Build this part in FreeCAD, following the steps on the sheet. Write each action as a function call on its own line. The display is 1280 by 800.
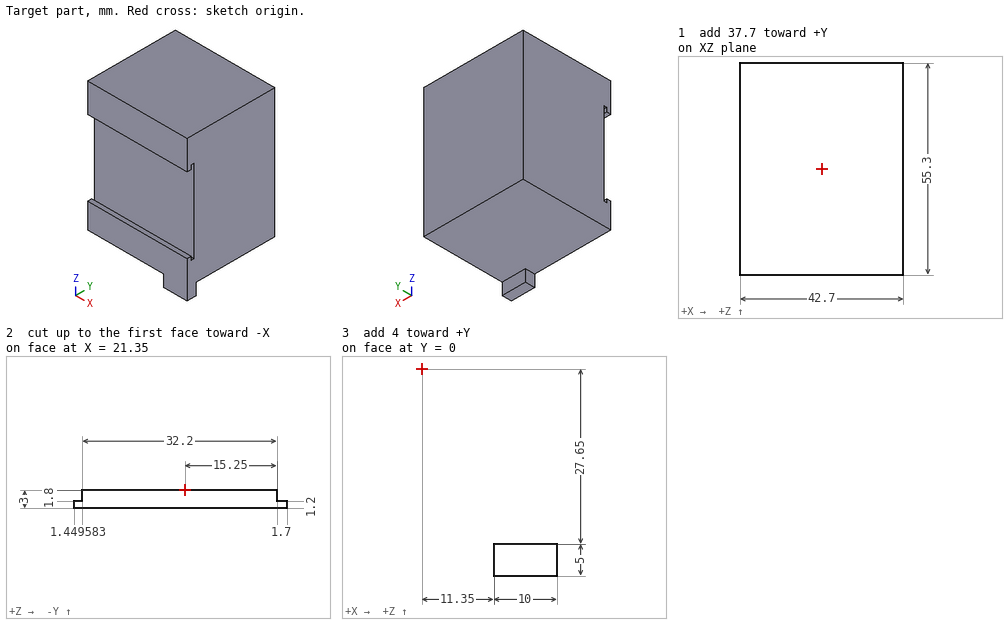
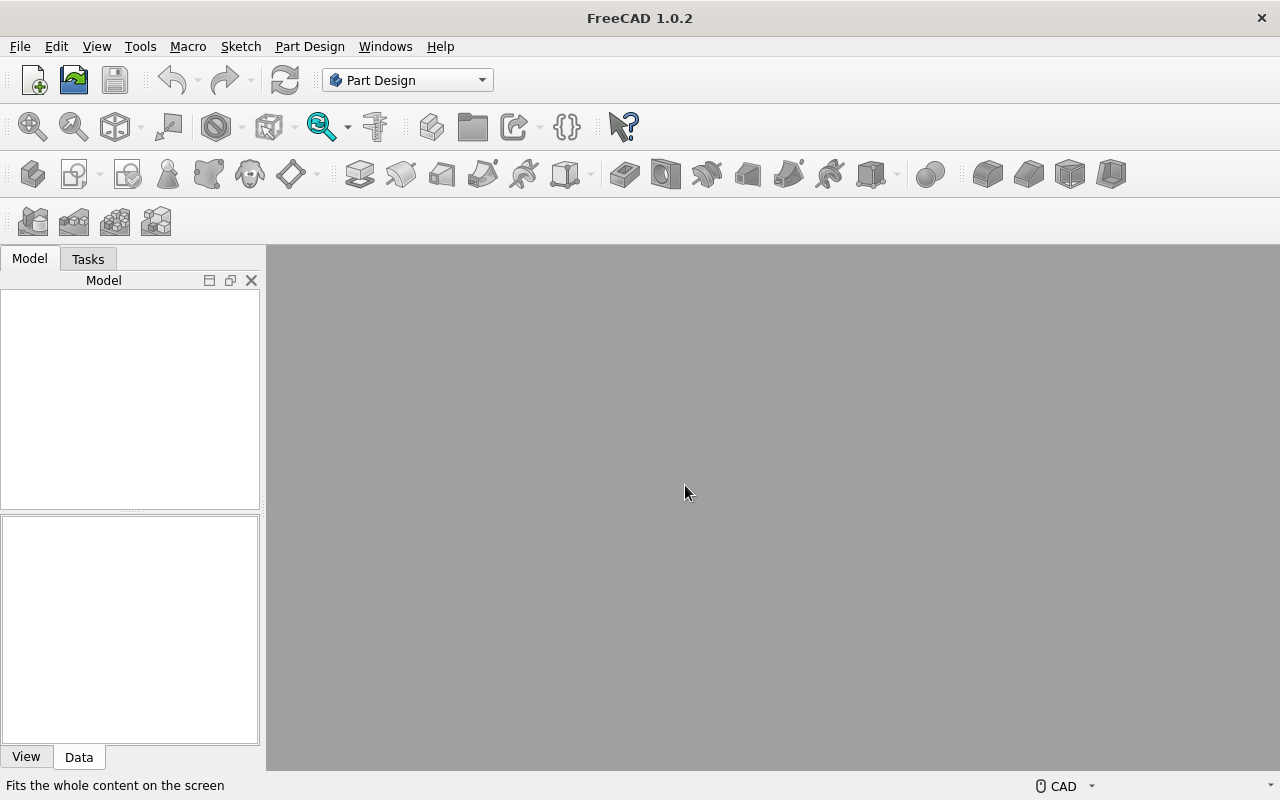
key(ctrl+n)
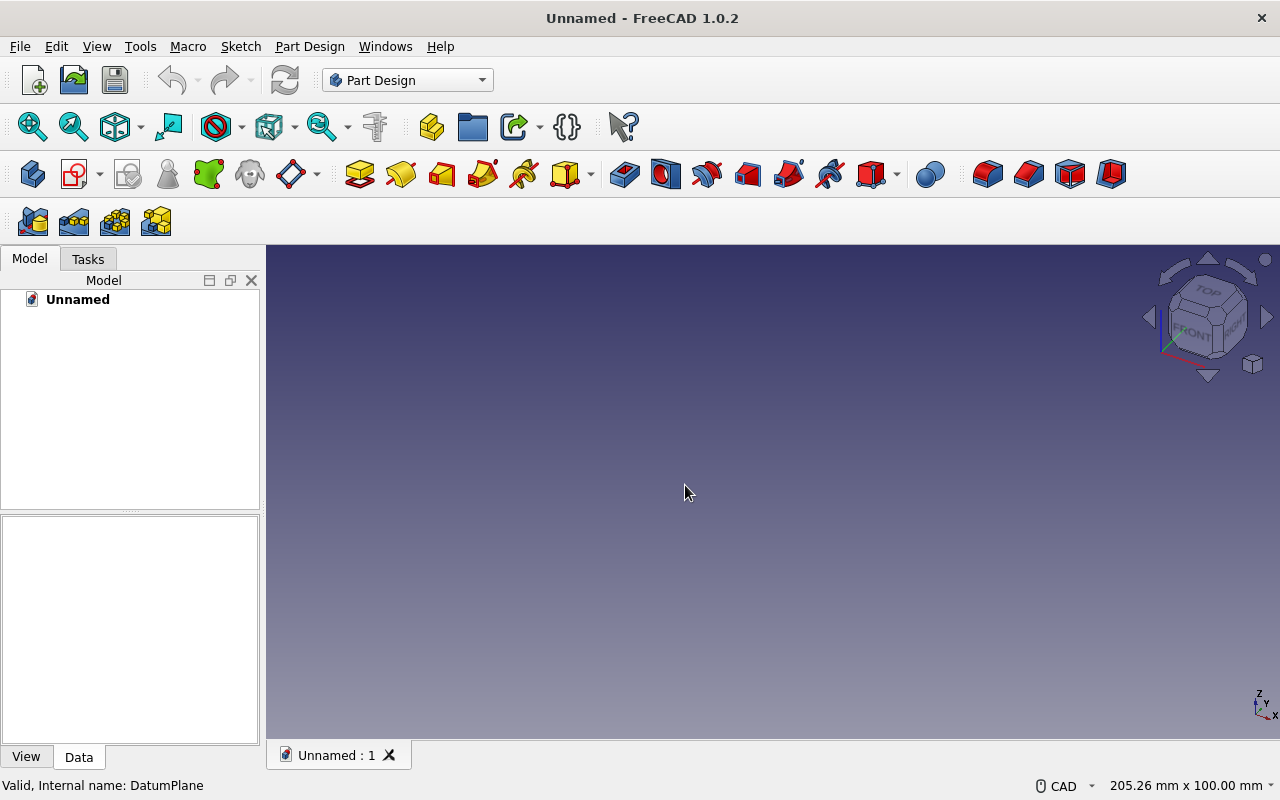
click(74, 174)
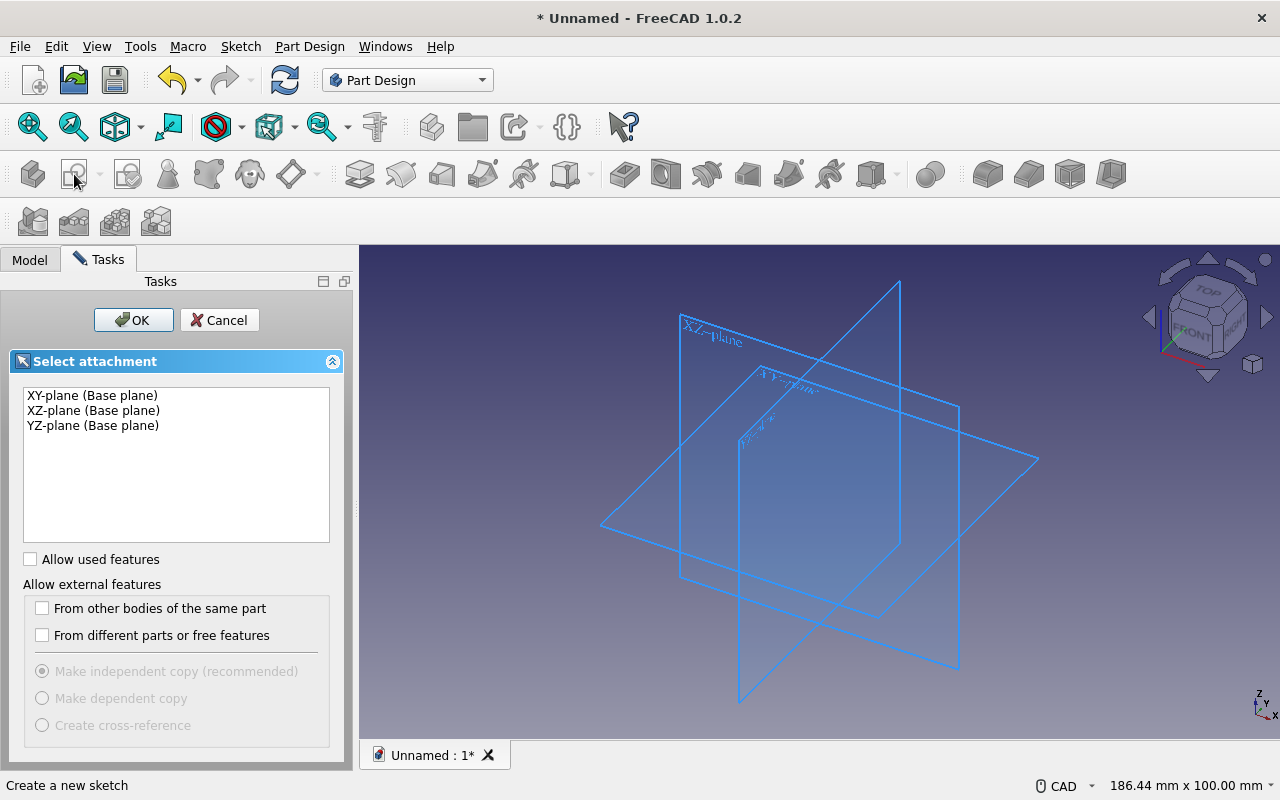
click(84, 410)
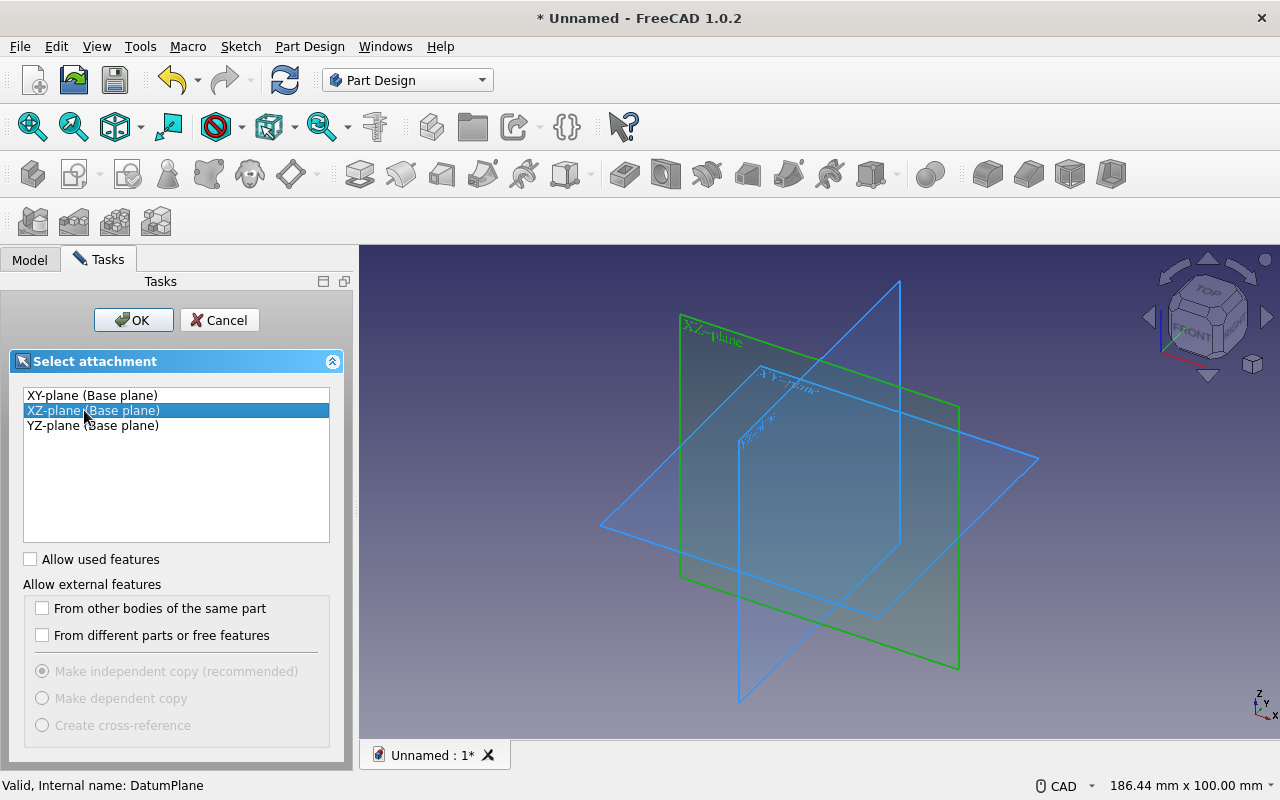
click(134, 320)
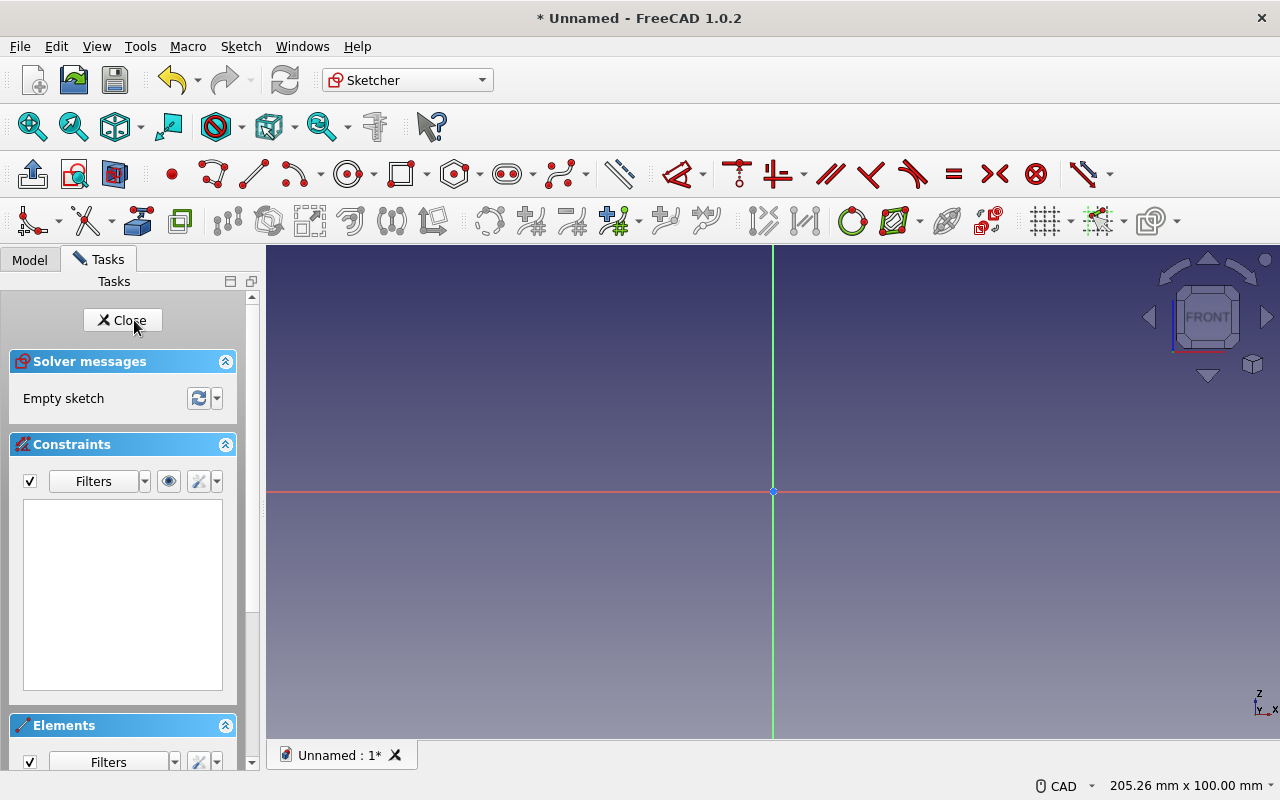
key(g)
key(v)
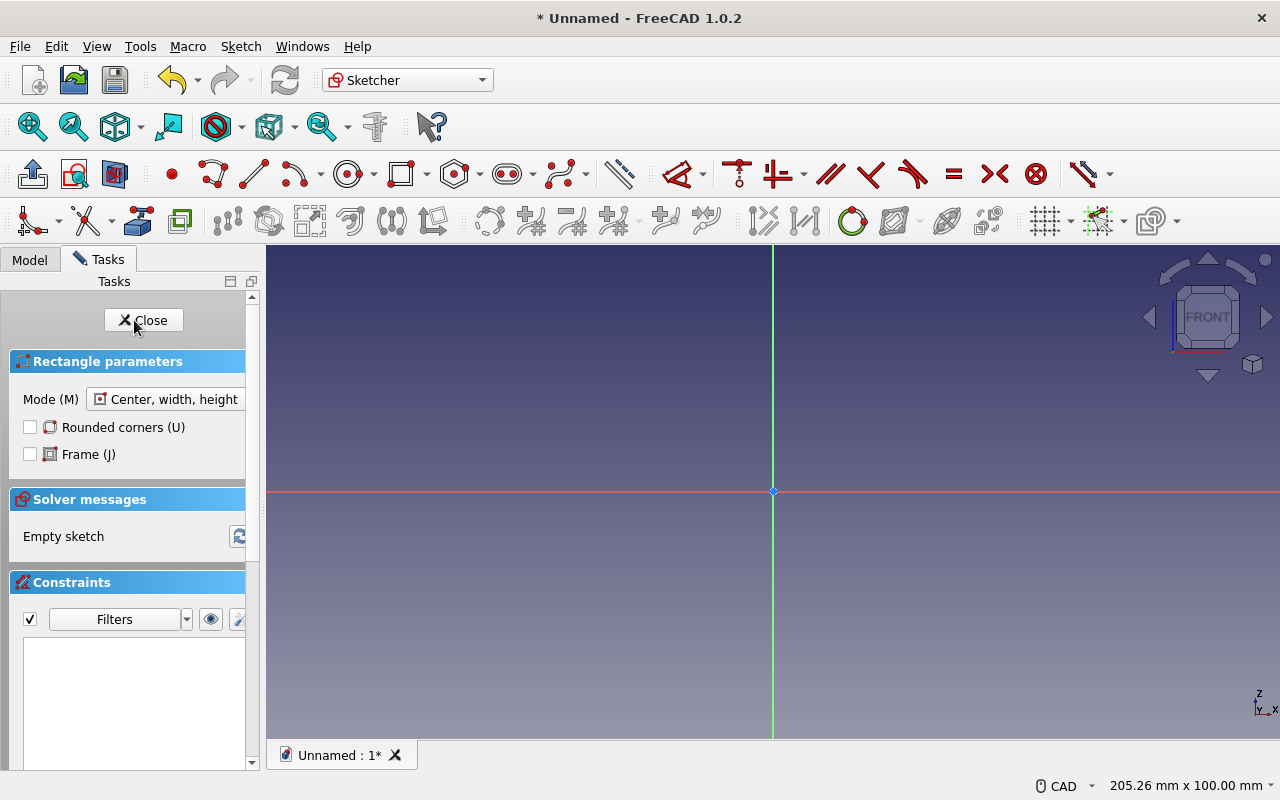
click(773, 492)
move(878, 355)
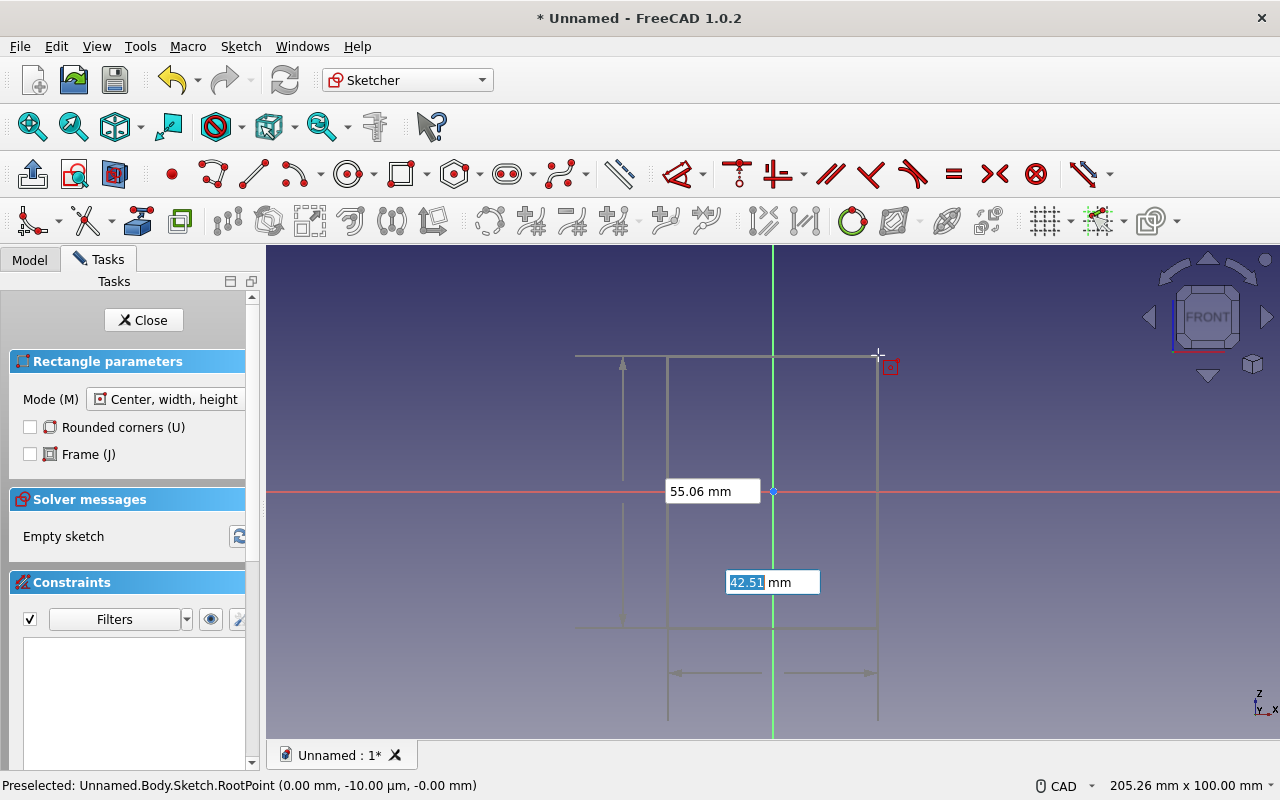
text(42.7)
key(Tab)
text(55.3)
key(Return)
key(Escape)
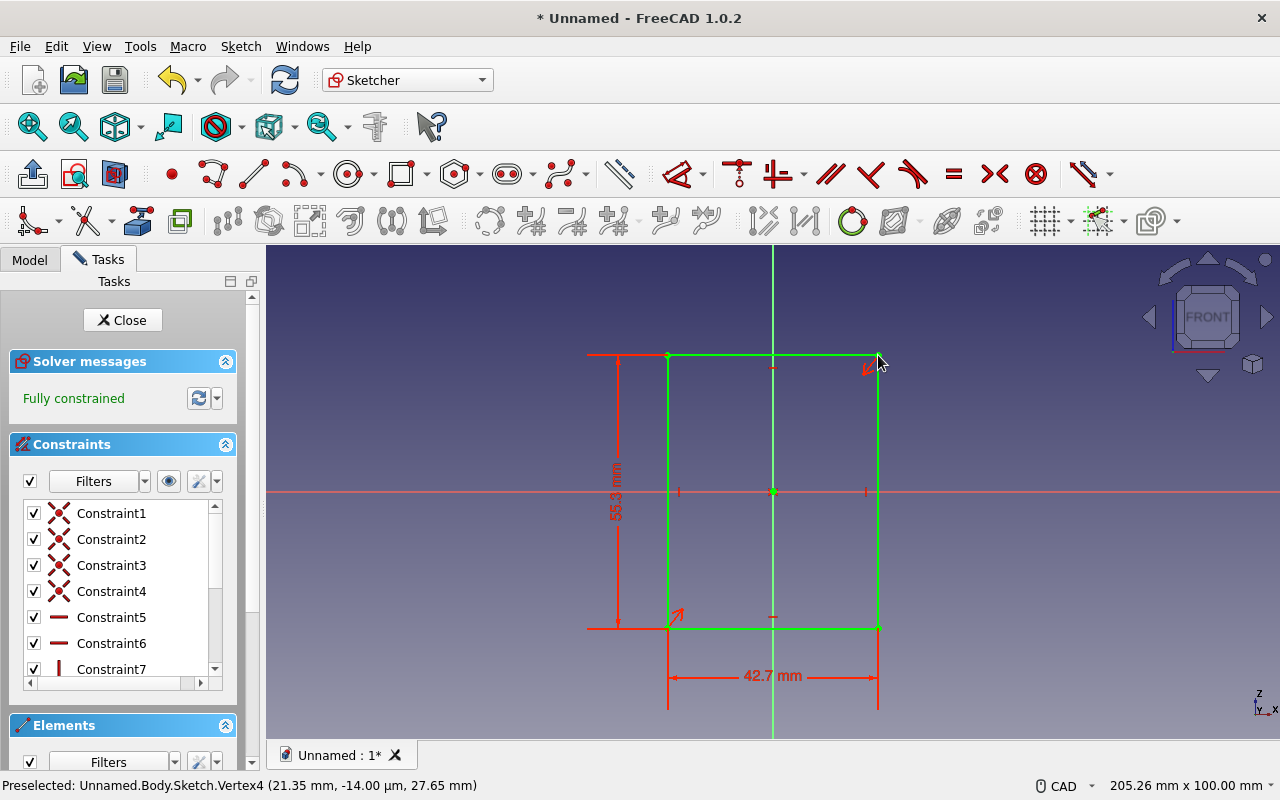
click(123, 320)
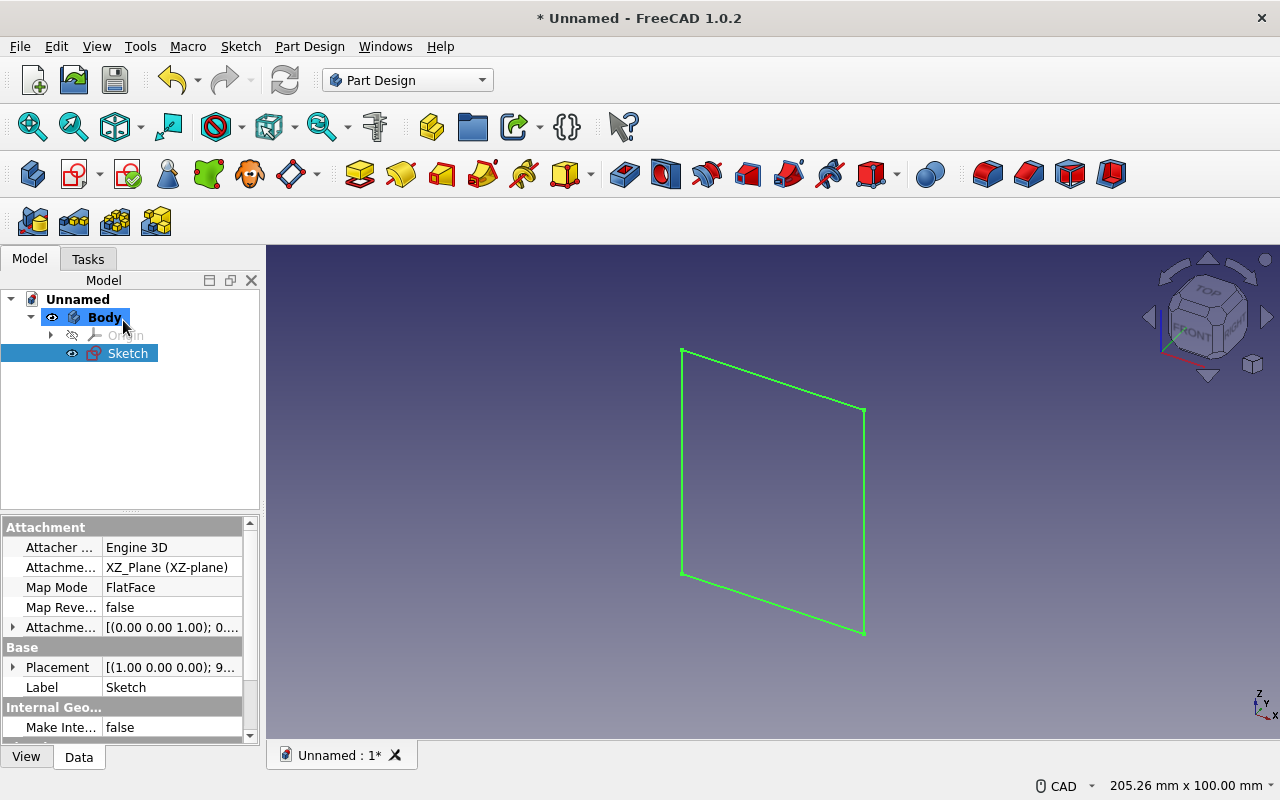
click(360, 174)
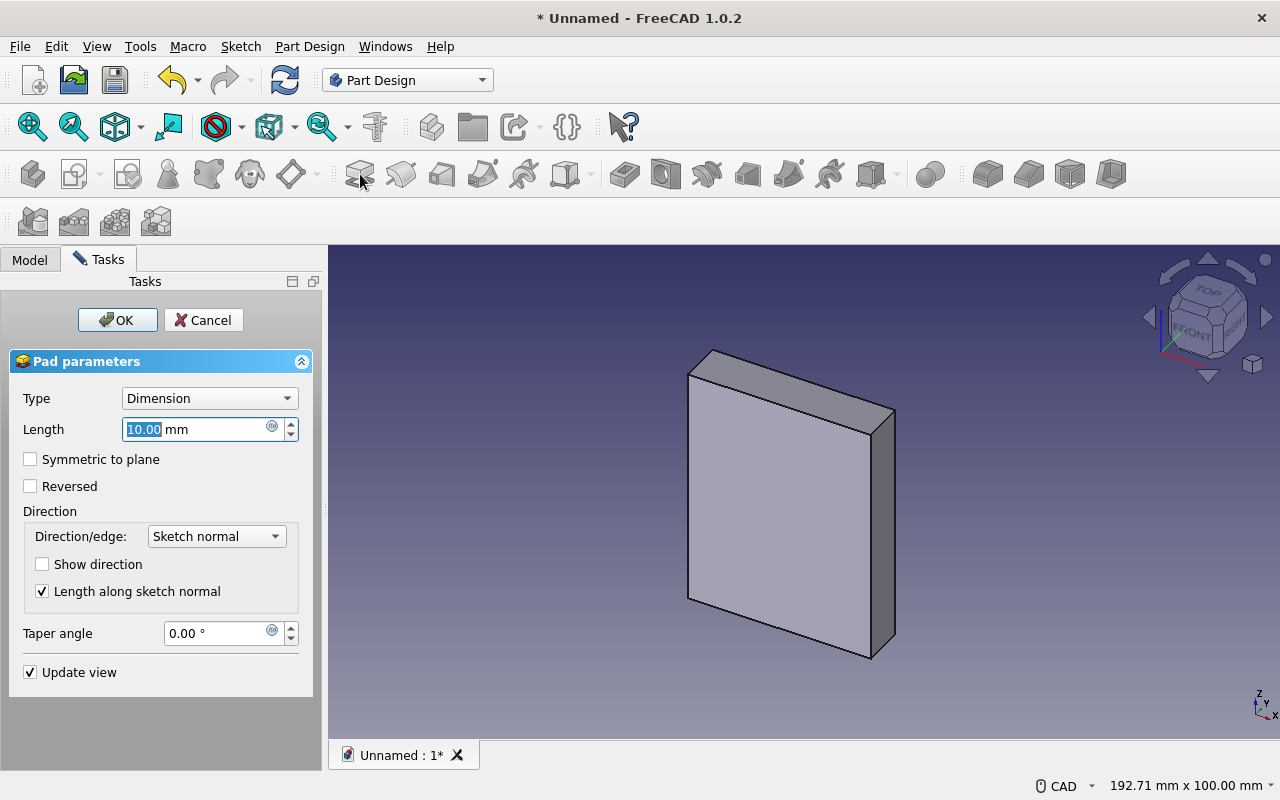
text(37.7)
key(Tab)